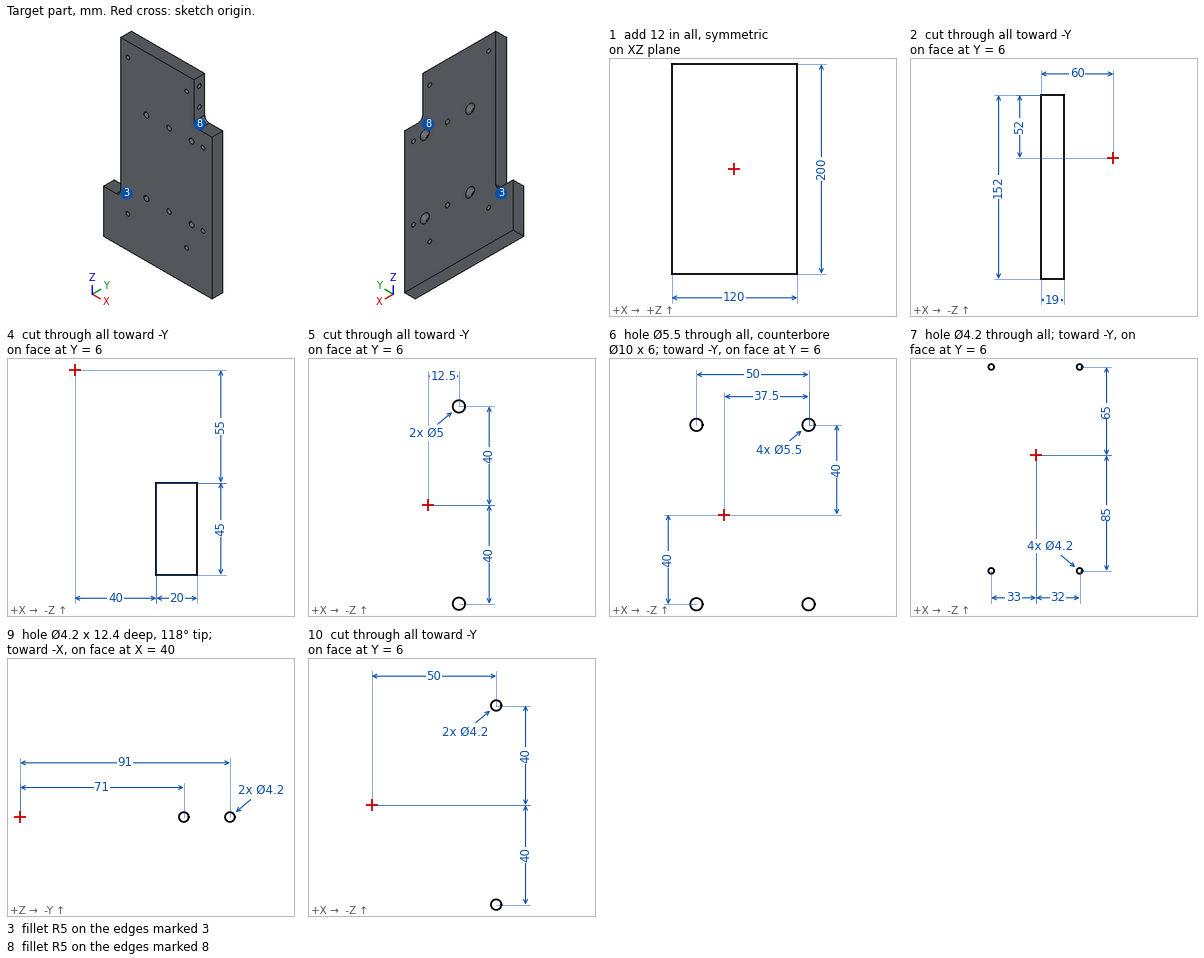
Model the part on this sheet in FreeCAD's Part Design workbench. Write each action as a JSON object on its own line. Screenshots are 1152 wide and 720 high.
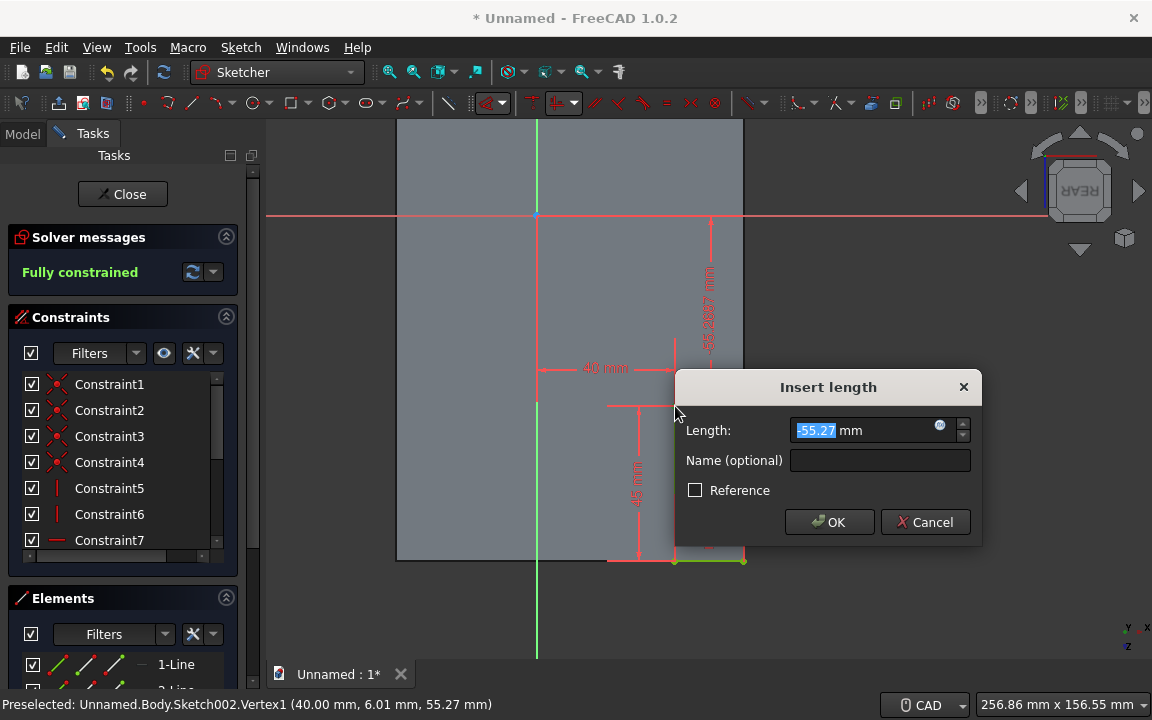
{"action": "type", "text": "-55"}
{"action": "key", "text": "Return"}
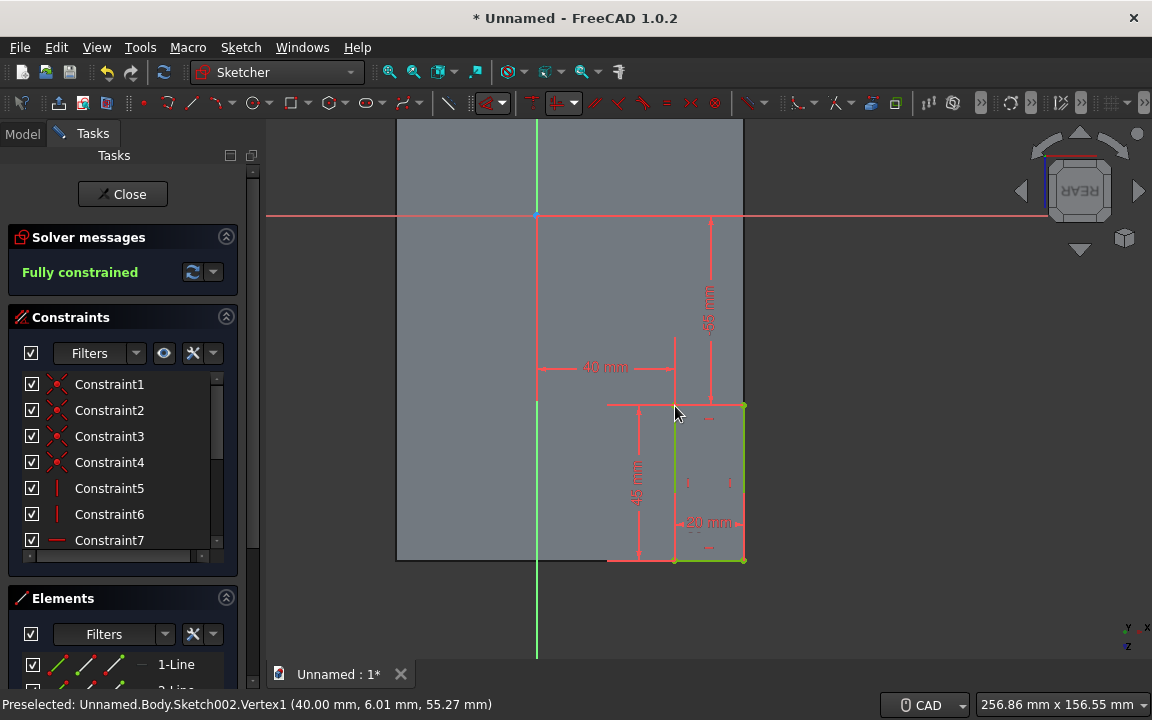
{"action": "left_click", "coordinate": [123, 194]}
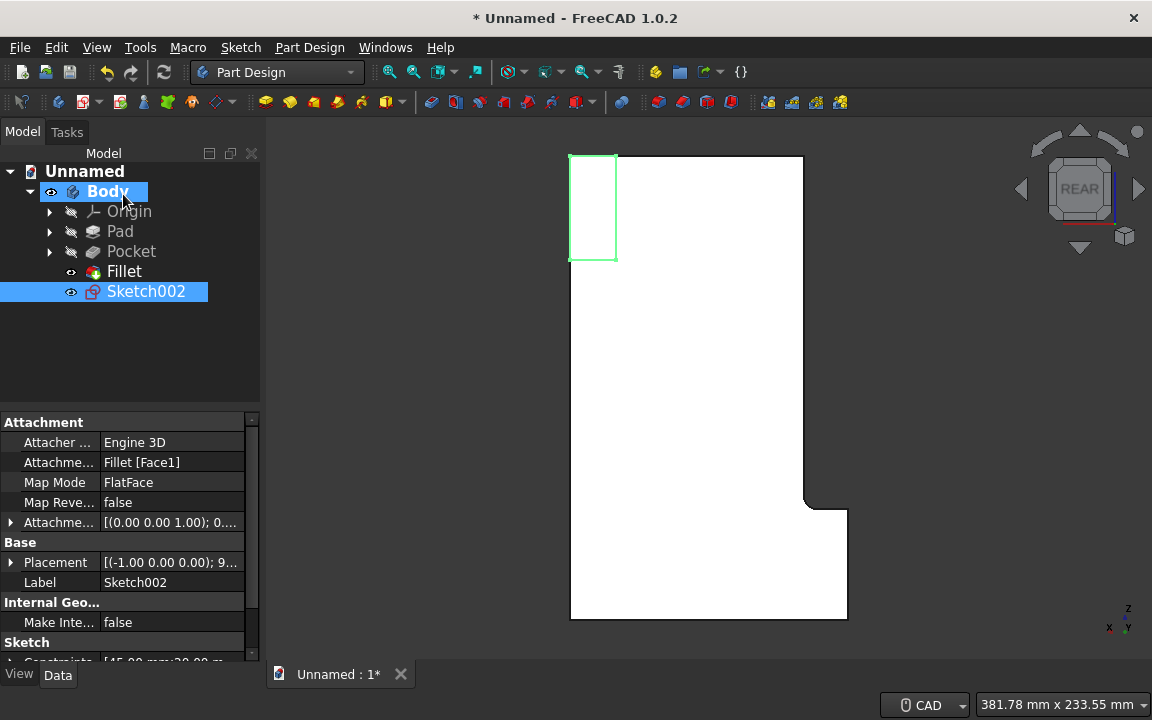
{"action": "left_click", "coordinate": [432, 102]}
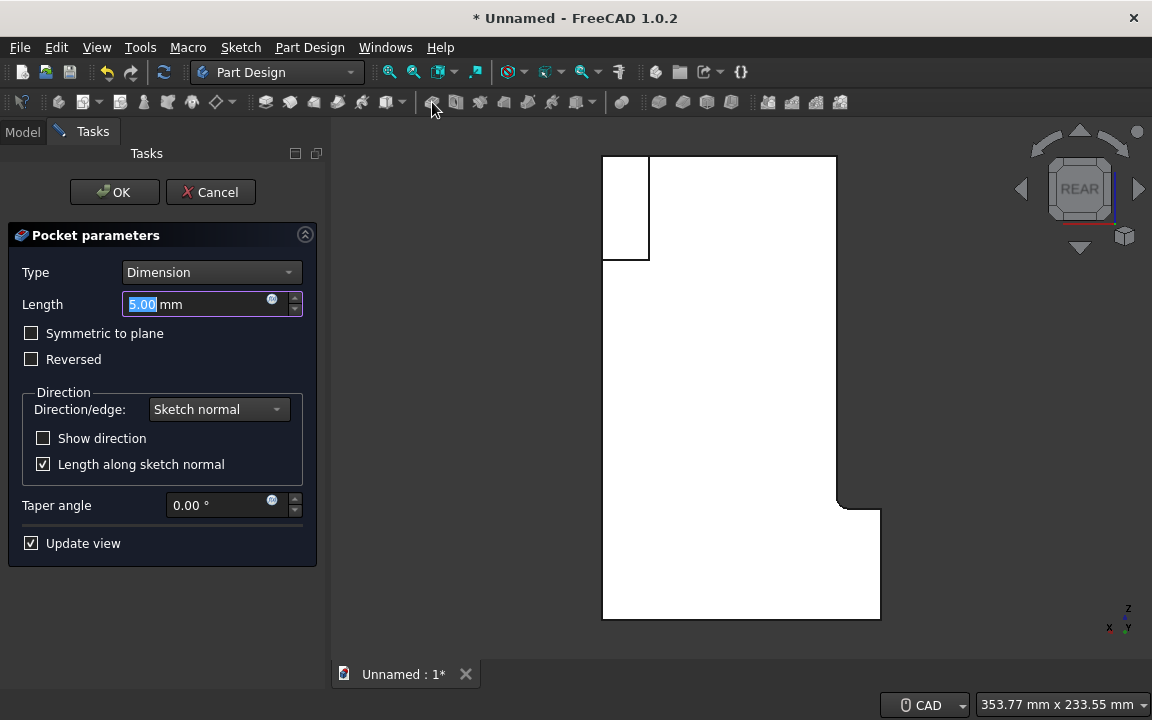
{"action": "left_click", "coordinate": [212, 272]}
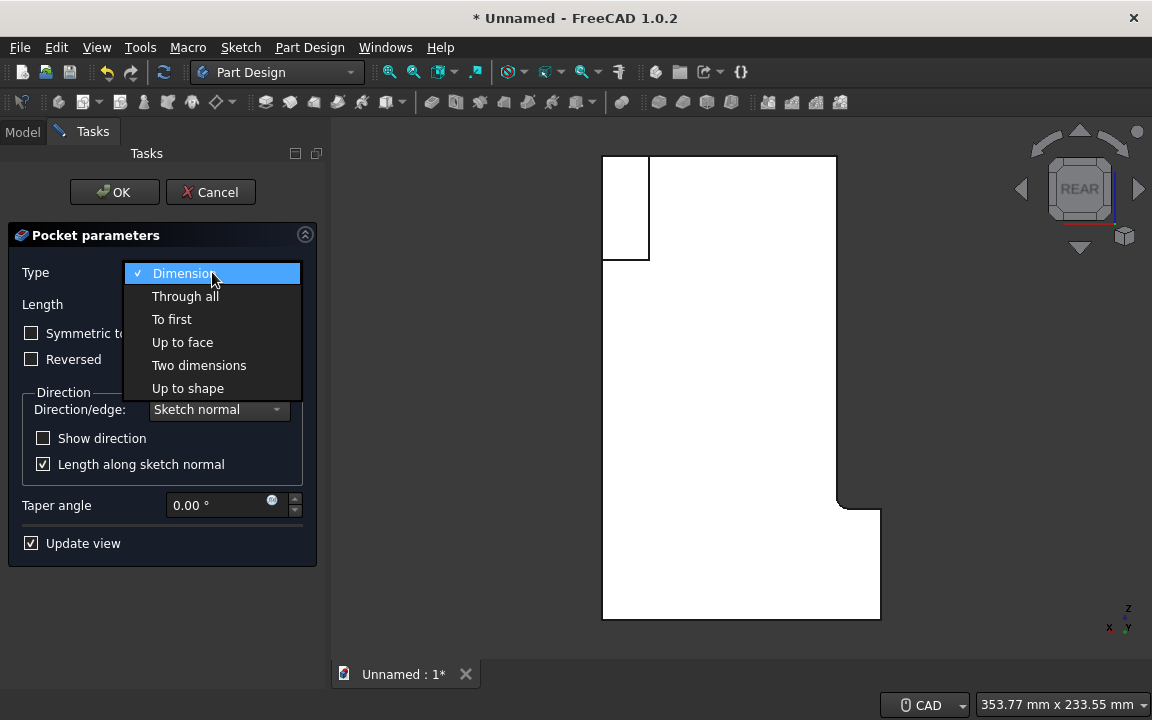
{"action": "left_click", "coordinate": [212, 296]}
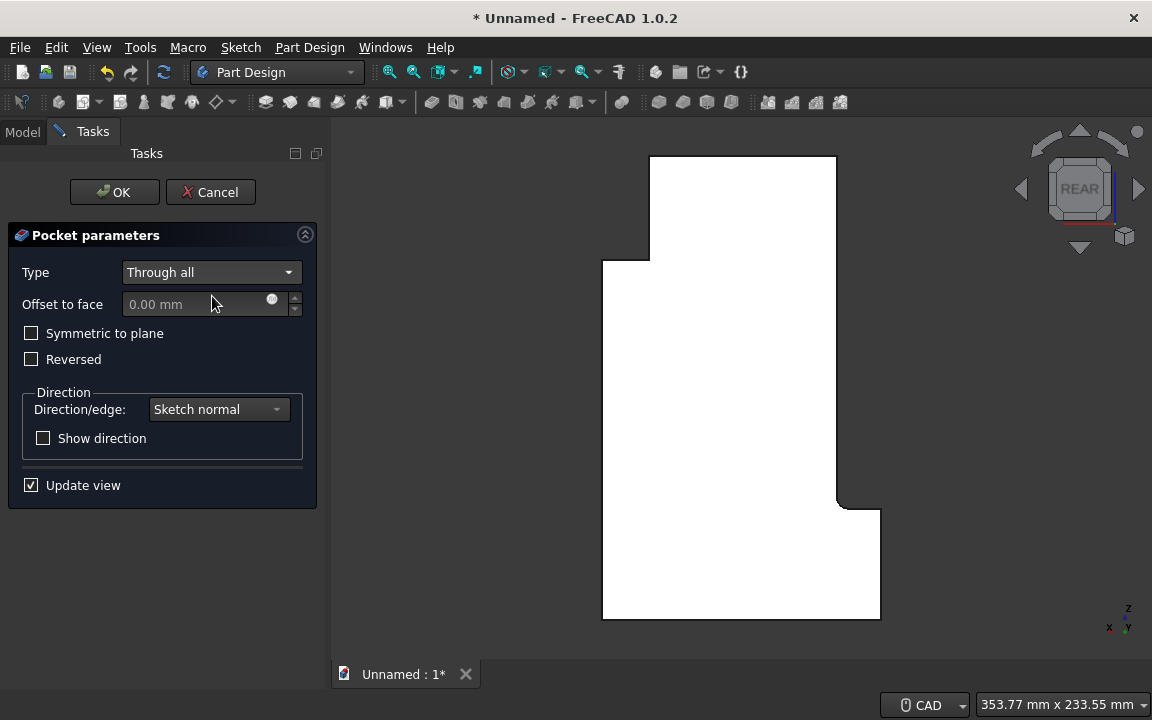
{"action": "left_click", "coordinate": [115, 192]}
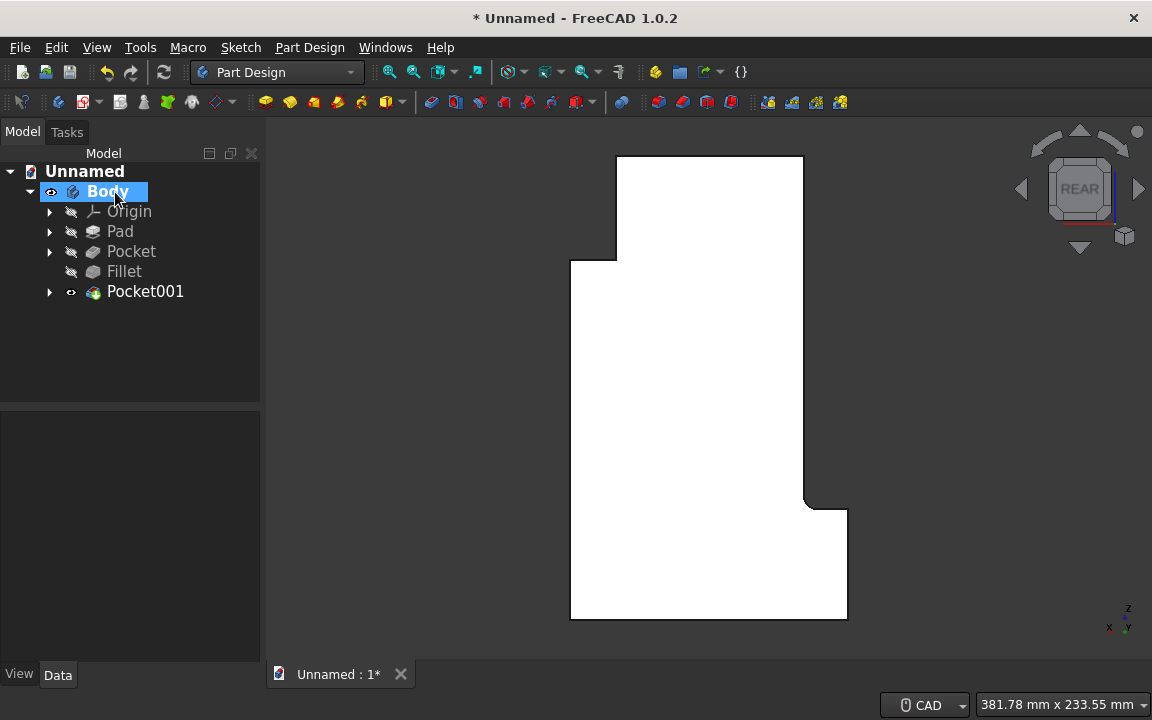
{"action": "left_click", "coordinate": [669, 387]}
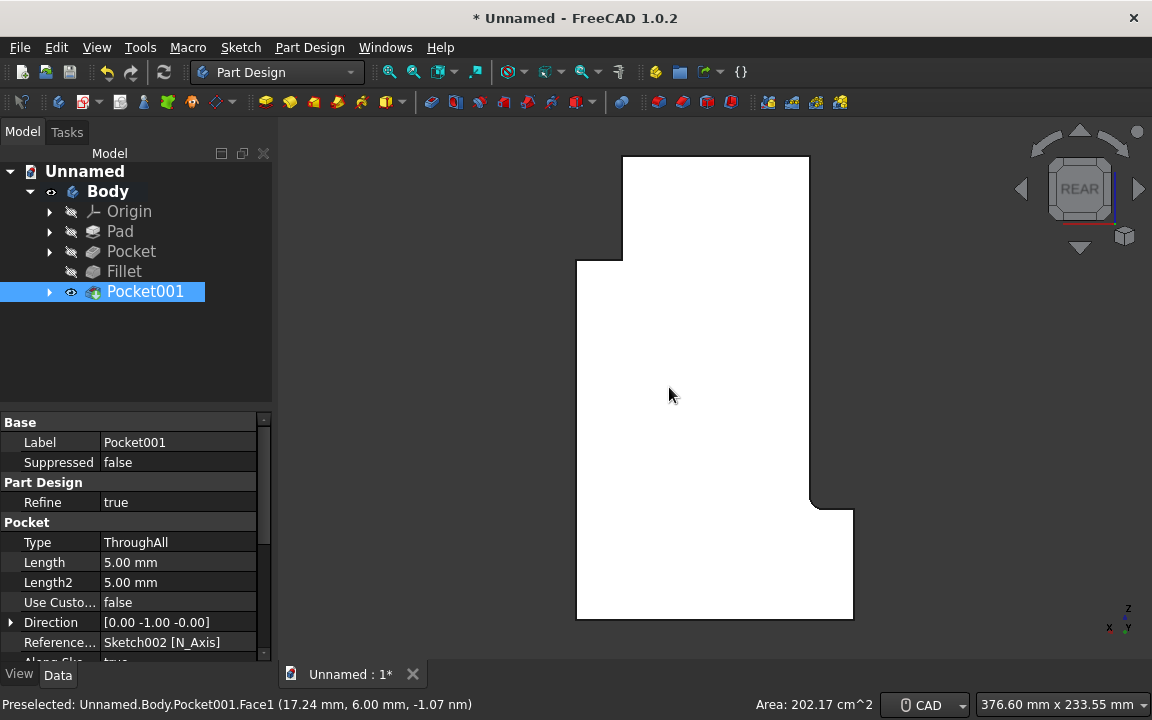
{"action": "left_click", "coordinate": [84, 102]}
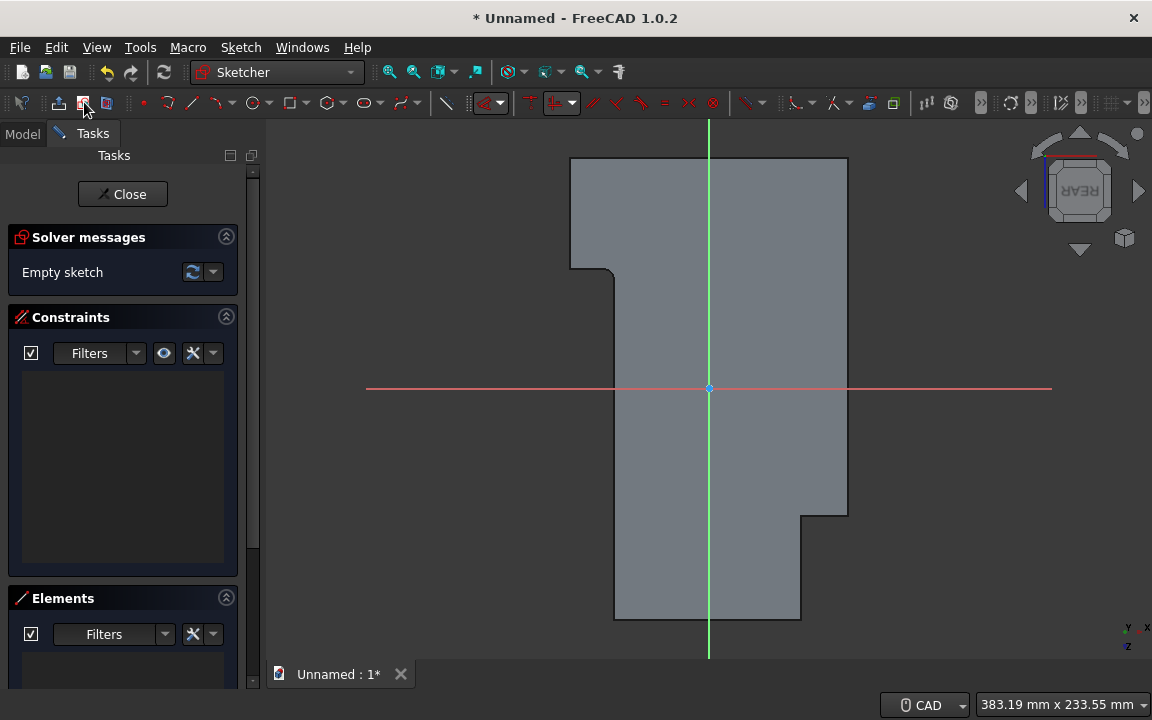
{"action": "scroll", "coordinate": [831, 389], "scroll_direction": "up", "scroll_amount": 3}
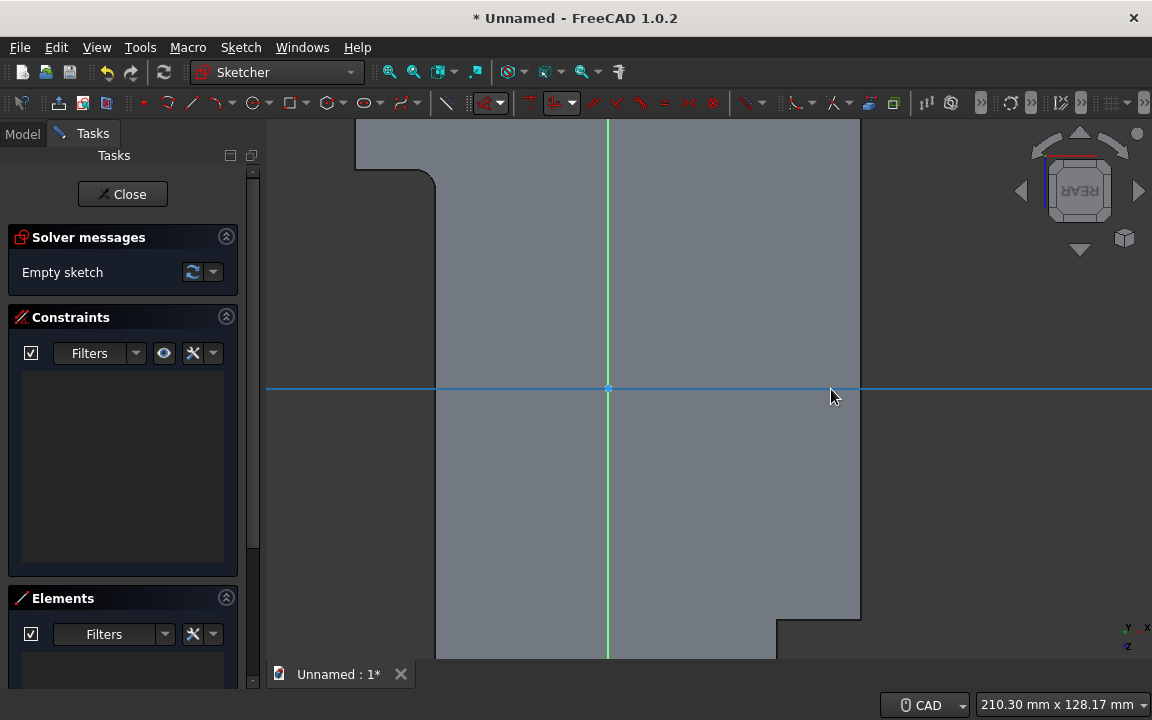
{"action": "left_click", "coordinate": [254, 104]}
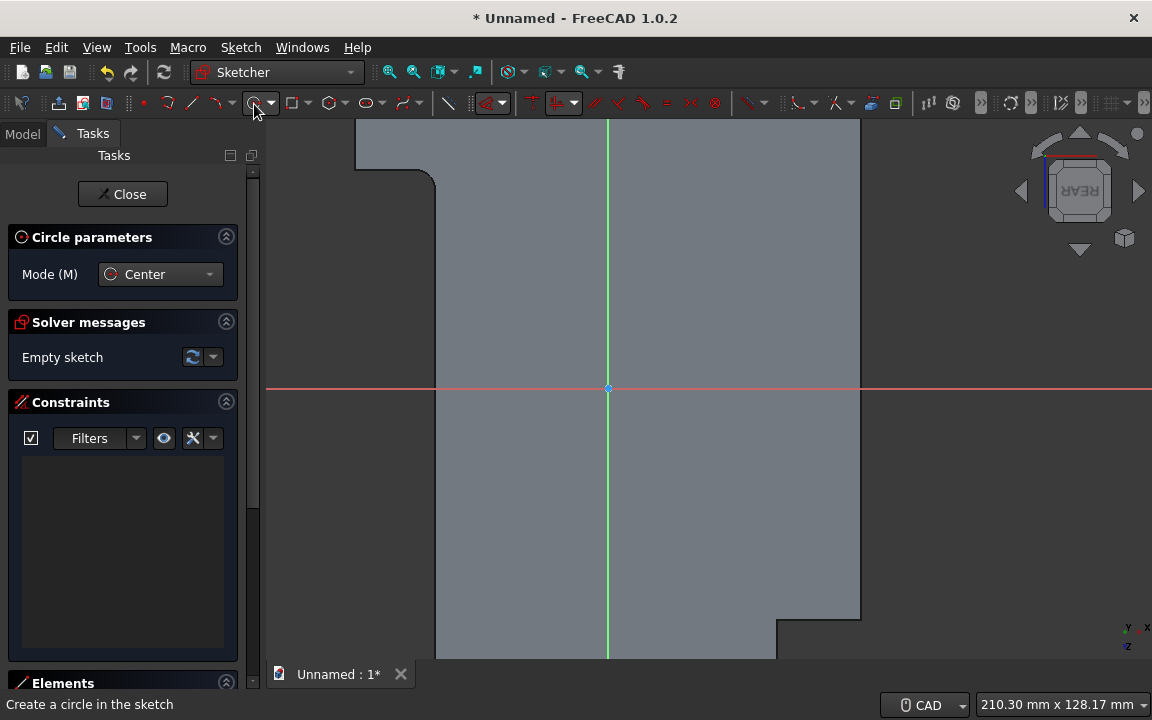
{"action": "scroll", "coordinate": [661, 220], "scroll_direction": "up", "scroll_amount": 4}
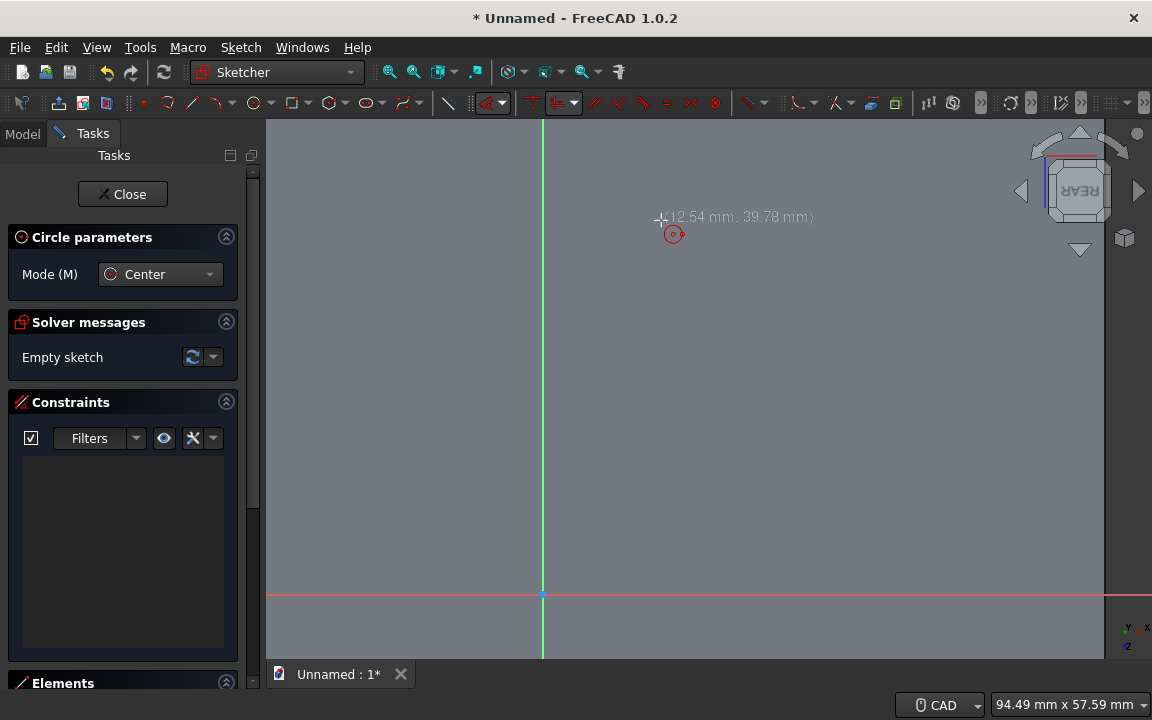
{"action": "left_click", "coordinate": [660, 220]}
{"action": "left_click", "coordinate": [677, 203]}